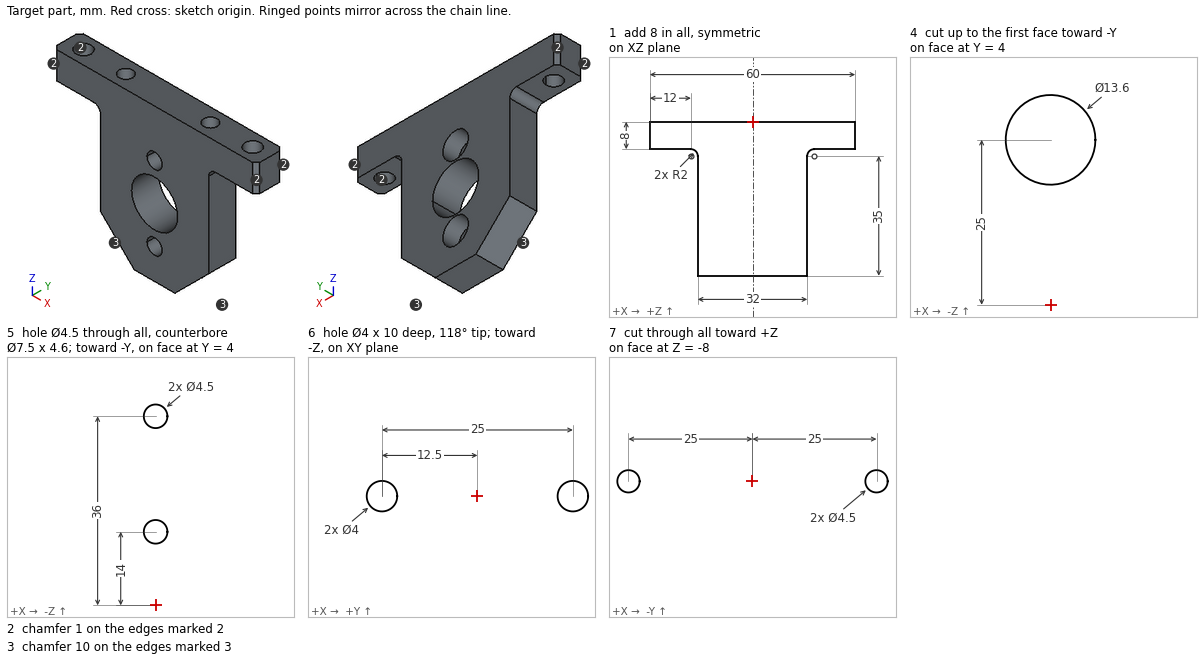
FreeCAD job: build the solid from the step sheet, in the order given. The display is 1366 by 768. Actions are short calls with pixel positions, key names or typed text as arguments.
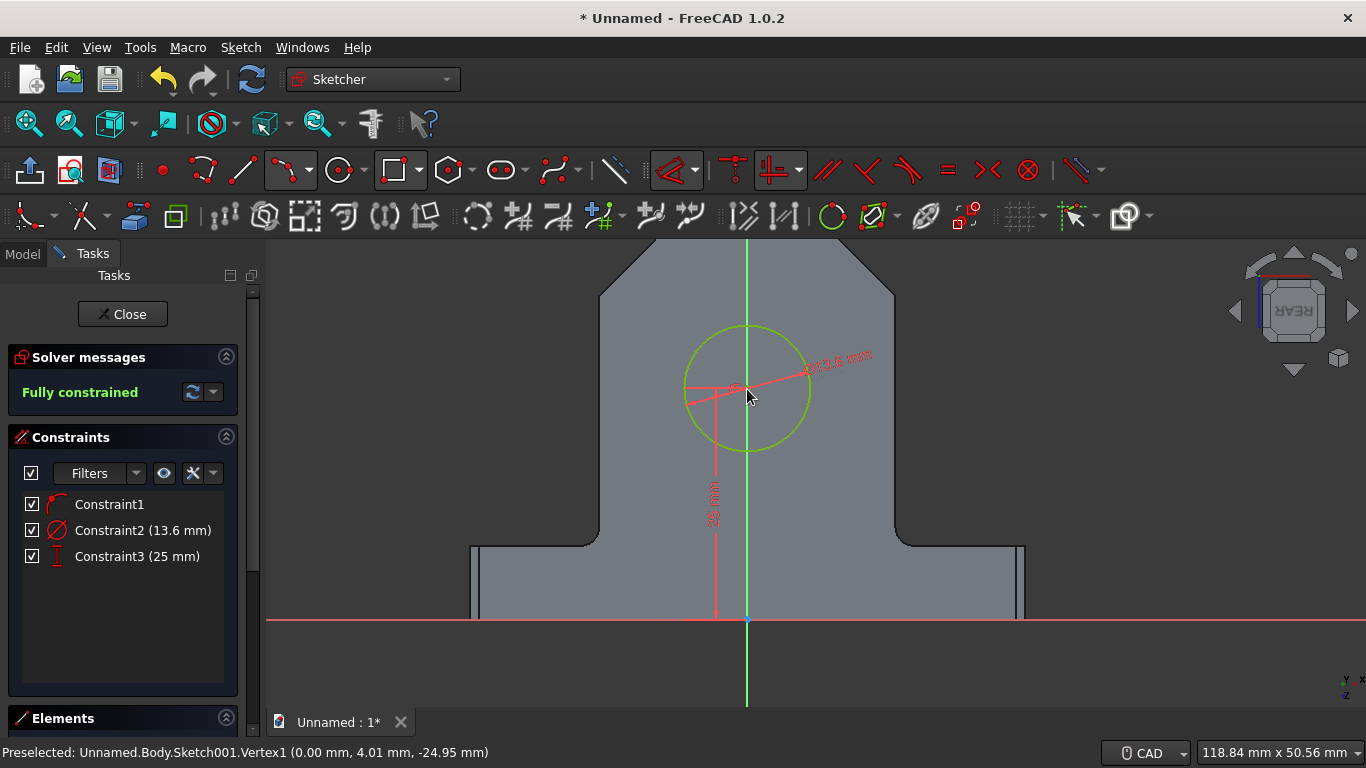
click(123, 314)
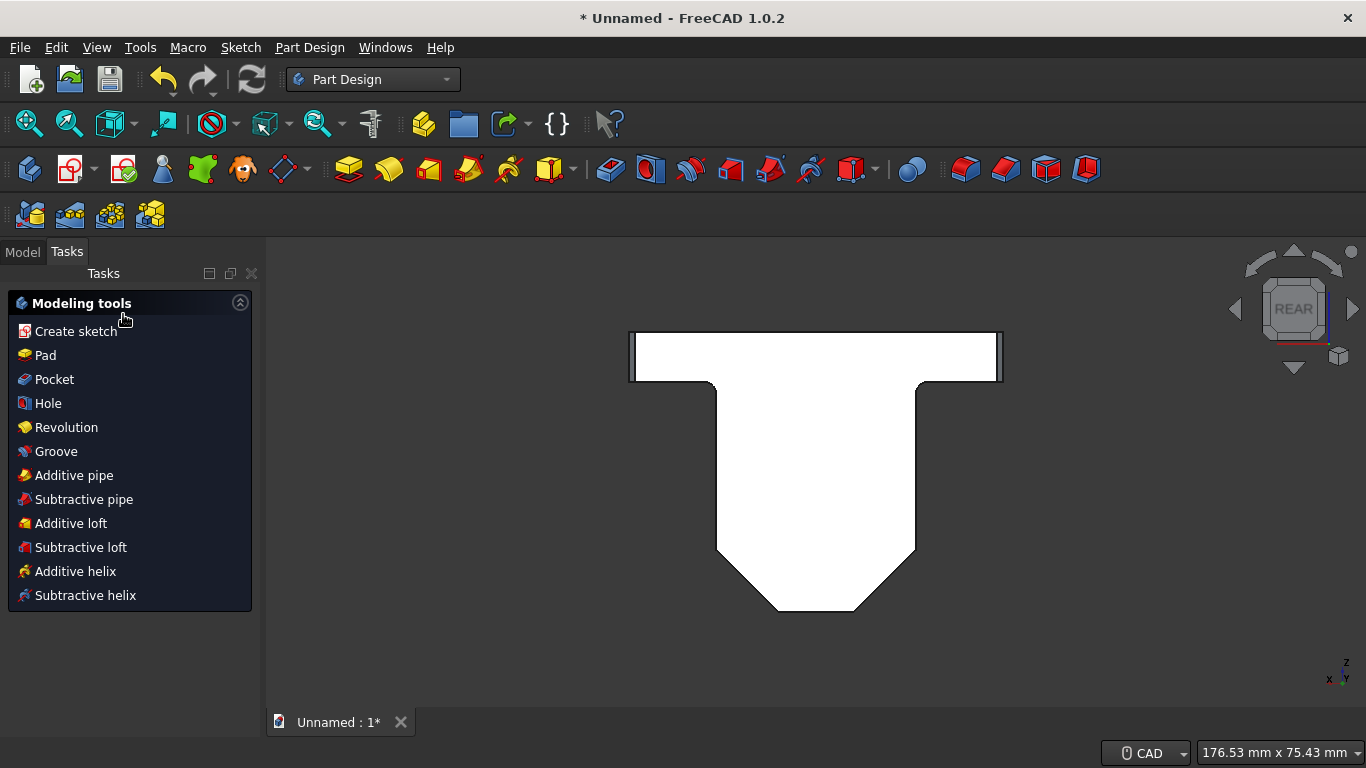
click(612, 170)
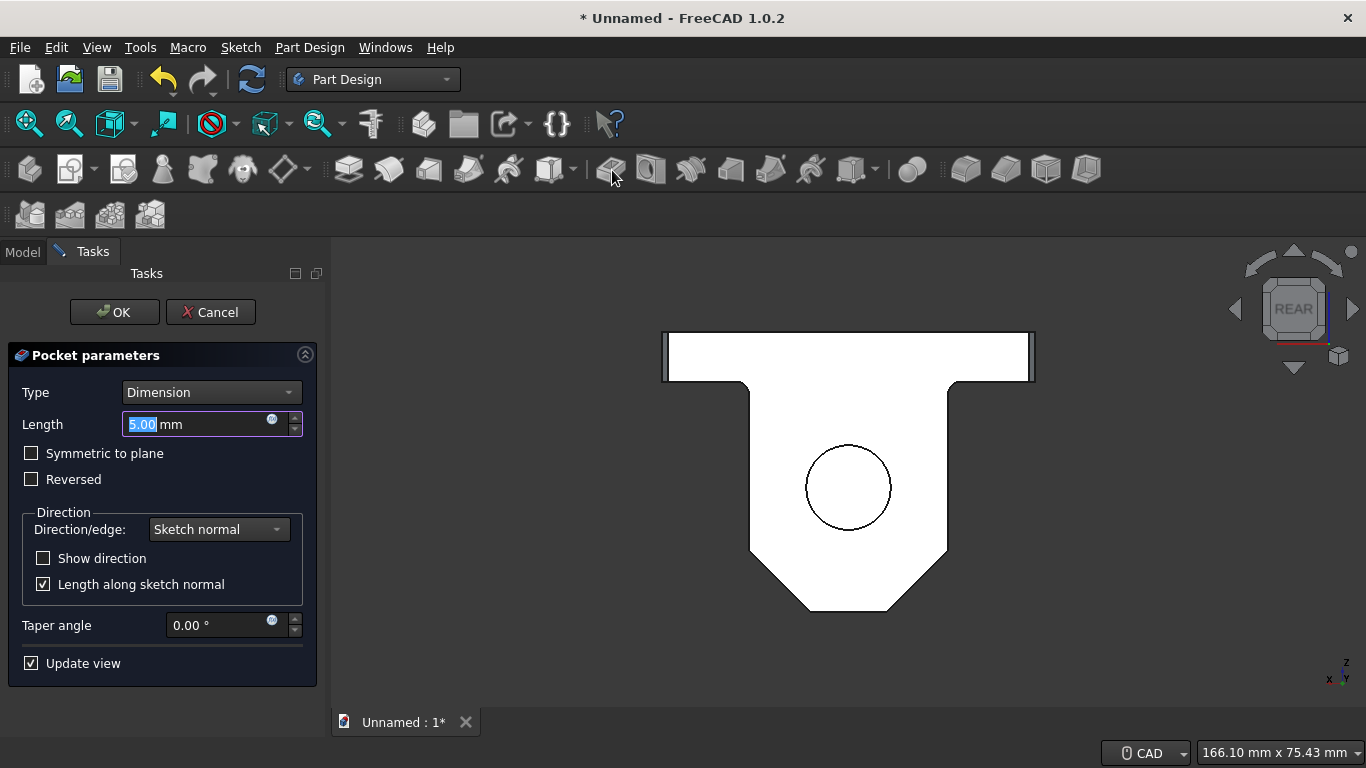
click(212, 392)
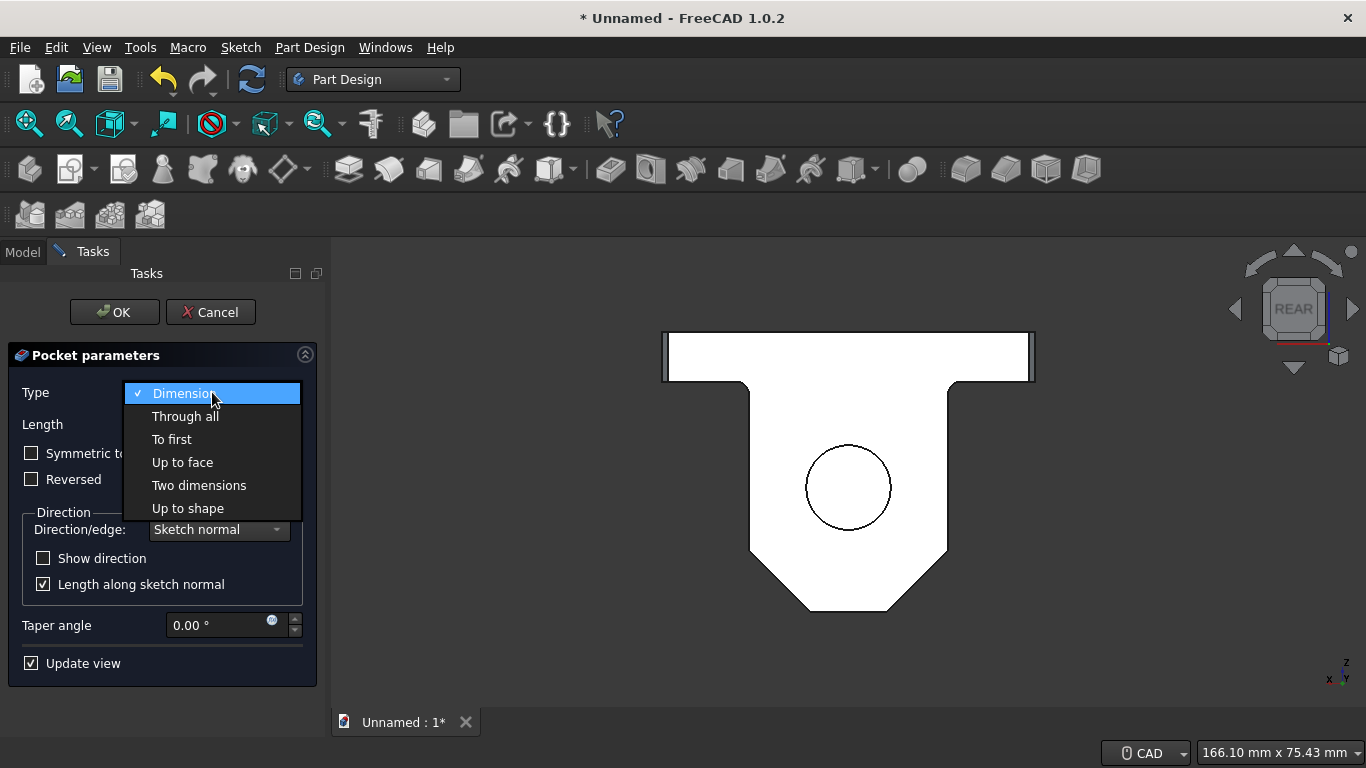
click(212, 440)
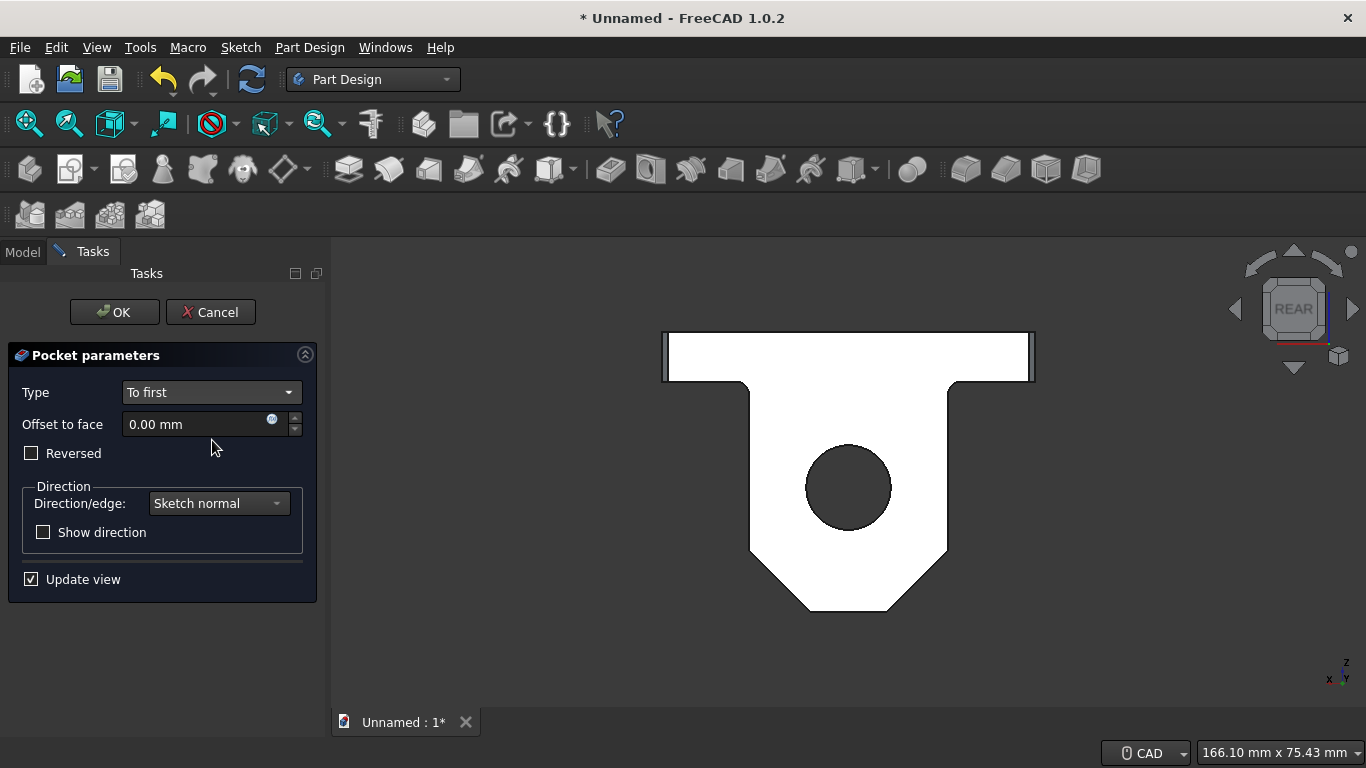
click(115, 312)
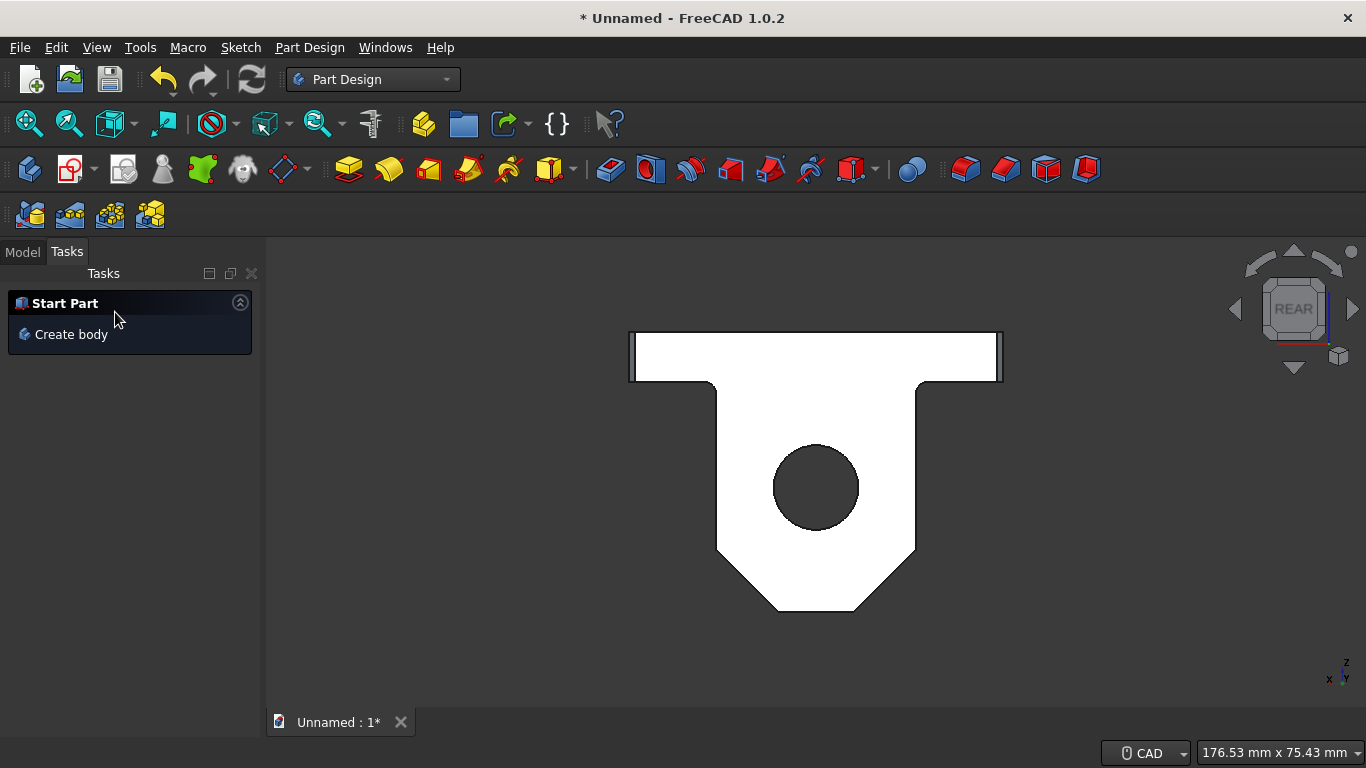
click(816, 391)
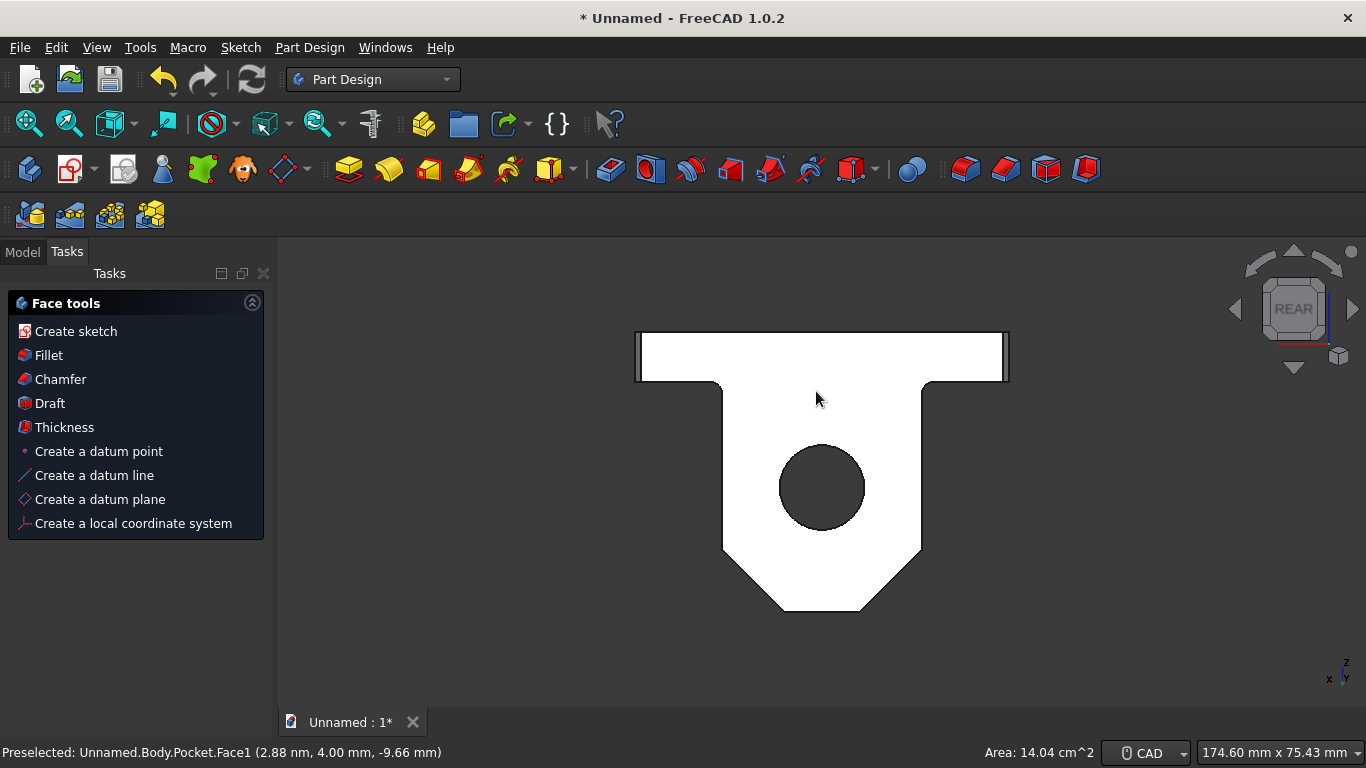
click(70, 170)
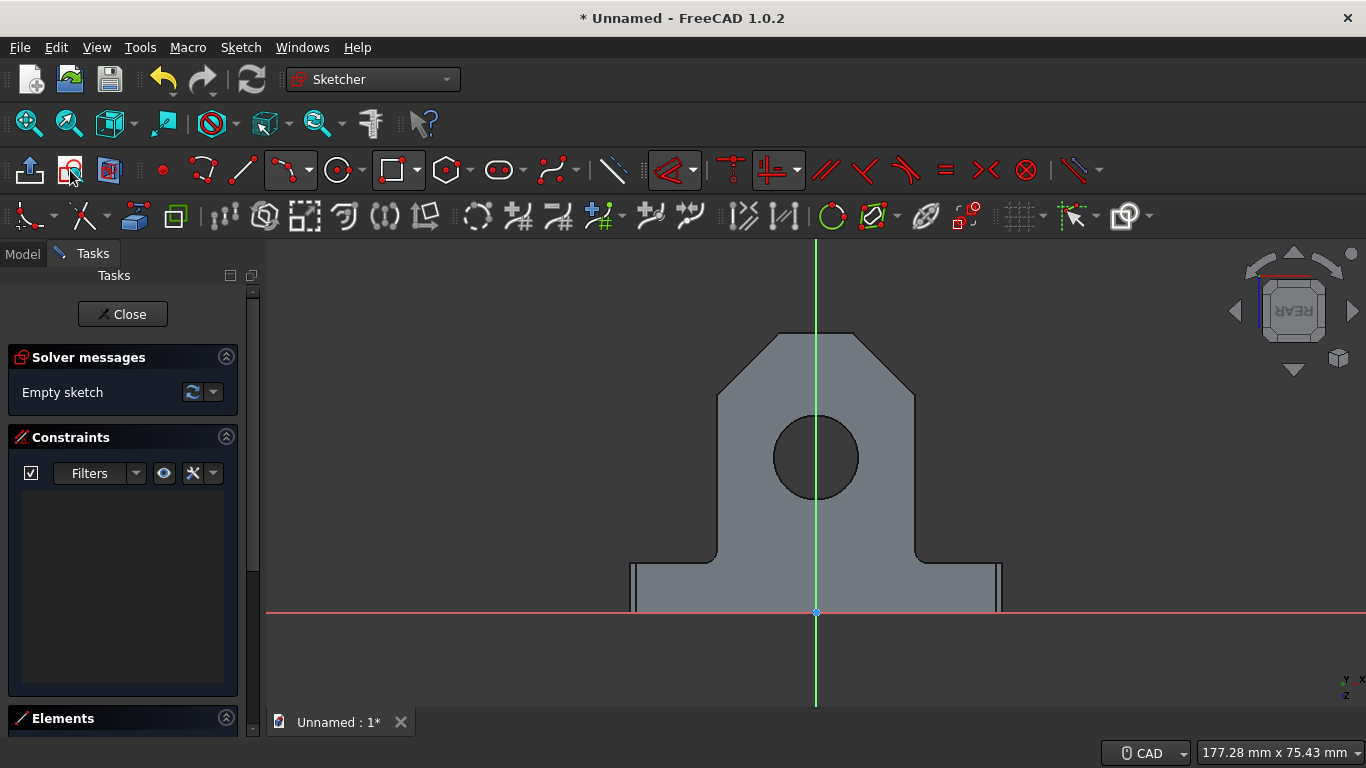
click(338, 170)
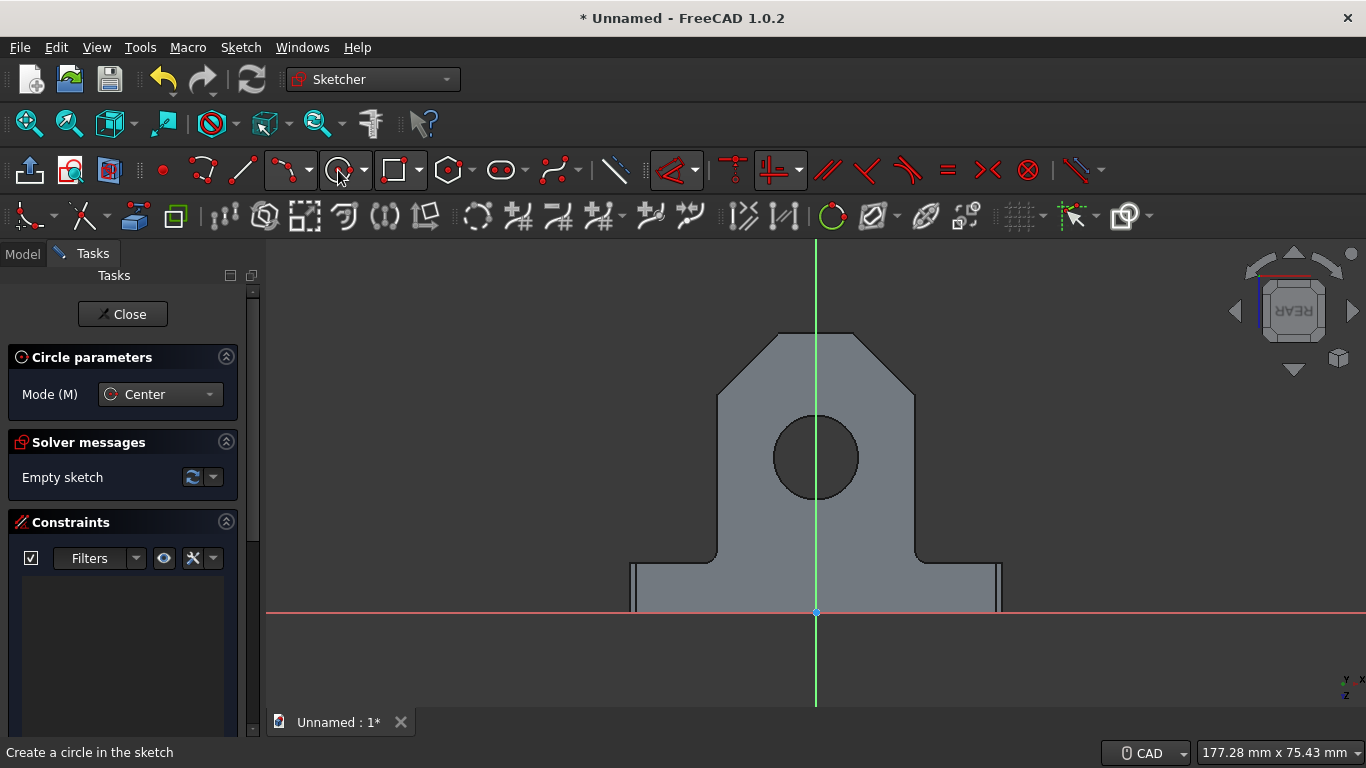
scroll(816, 389, up, 3)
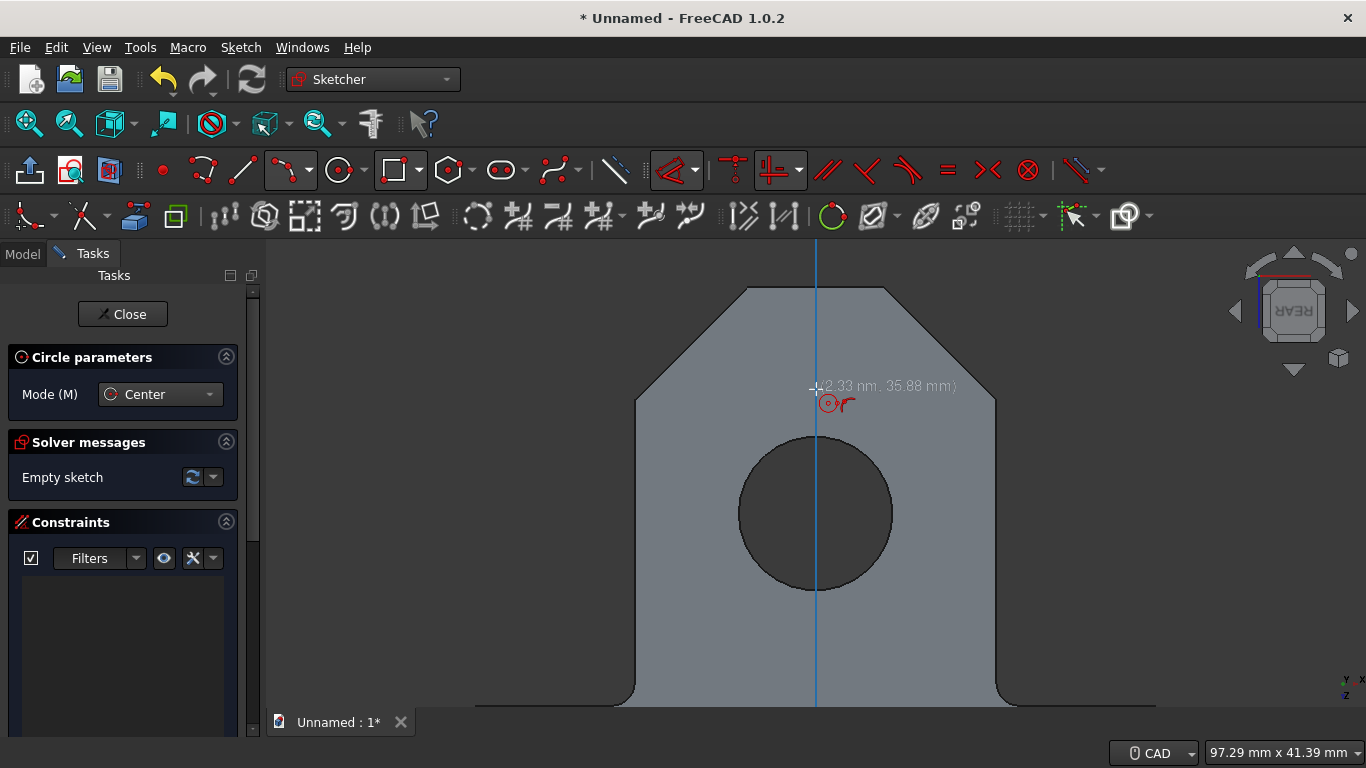
click(816, 389)
click(834, 371)